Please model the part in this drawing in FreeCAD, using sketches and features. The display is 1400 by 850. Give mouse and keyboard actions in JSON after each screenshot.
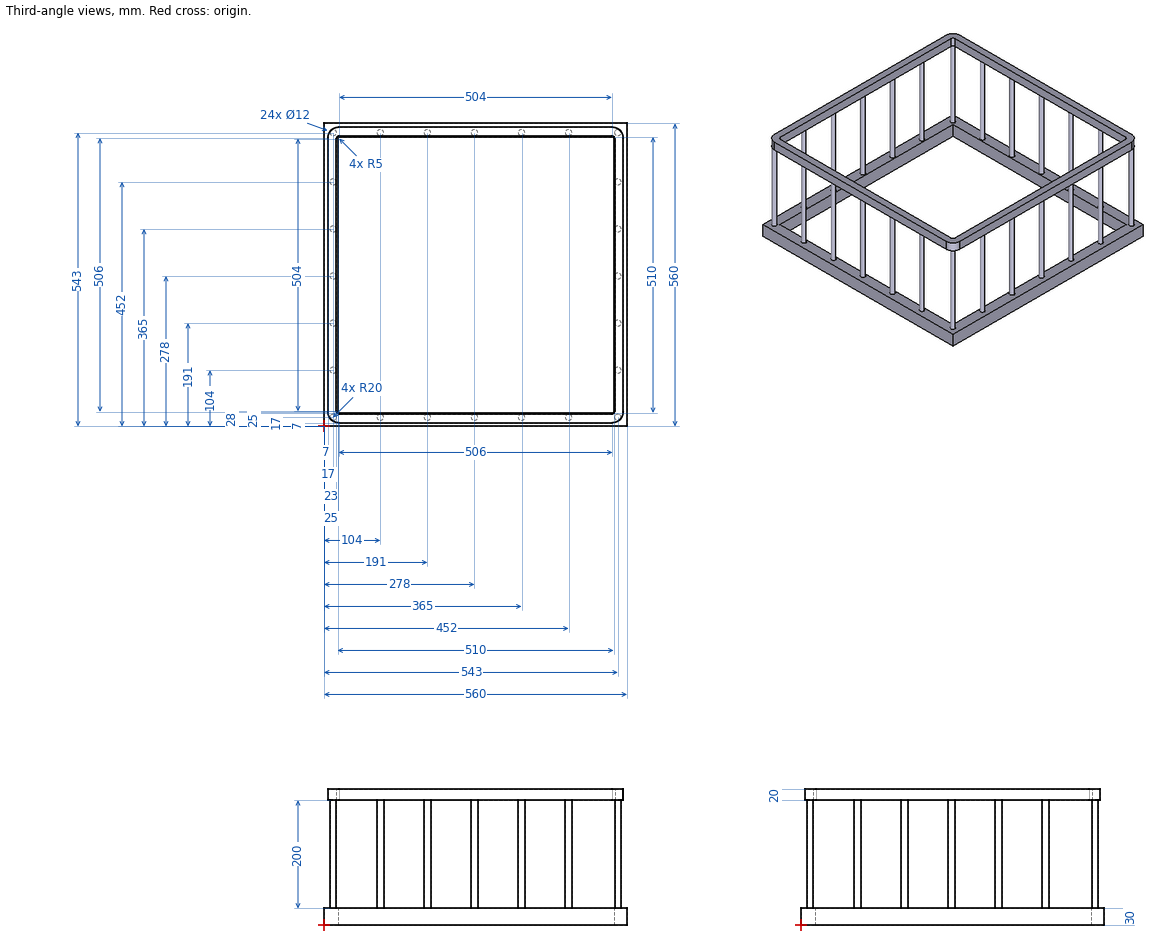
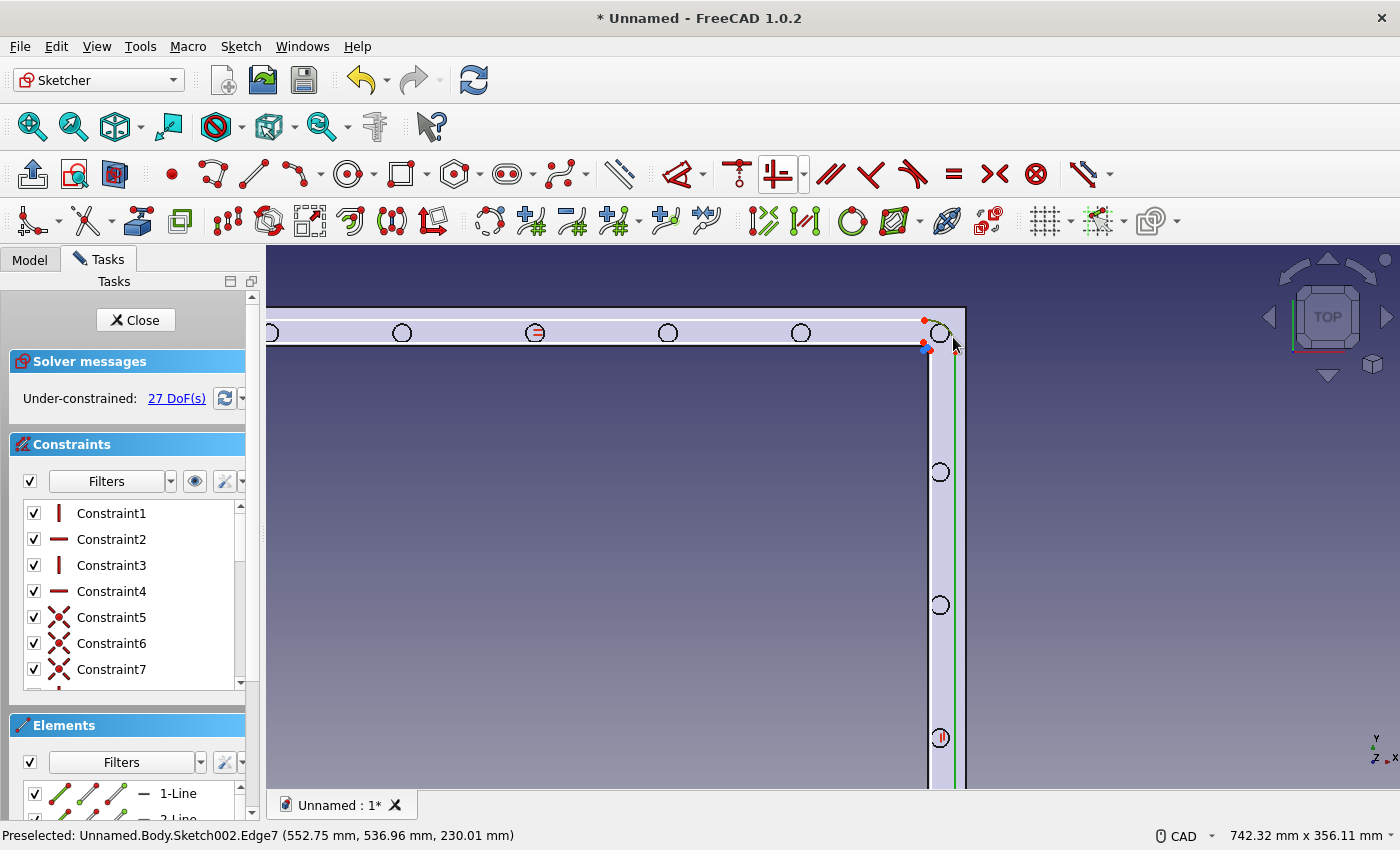
{"action": "left_click", "coordinate": [913, 174]}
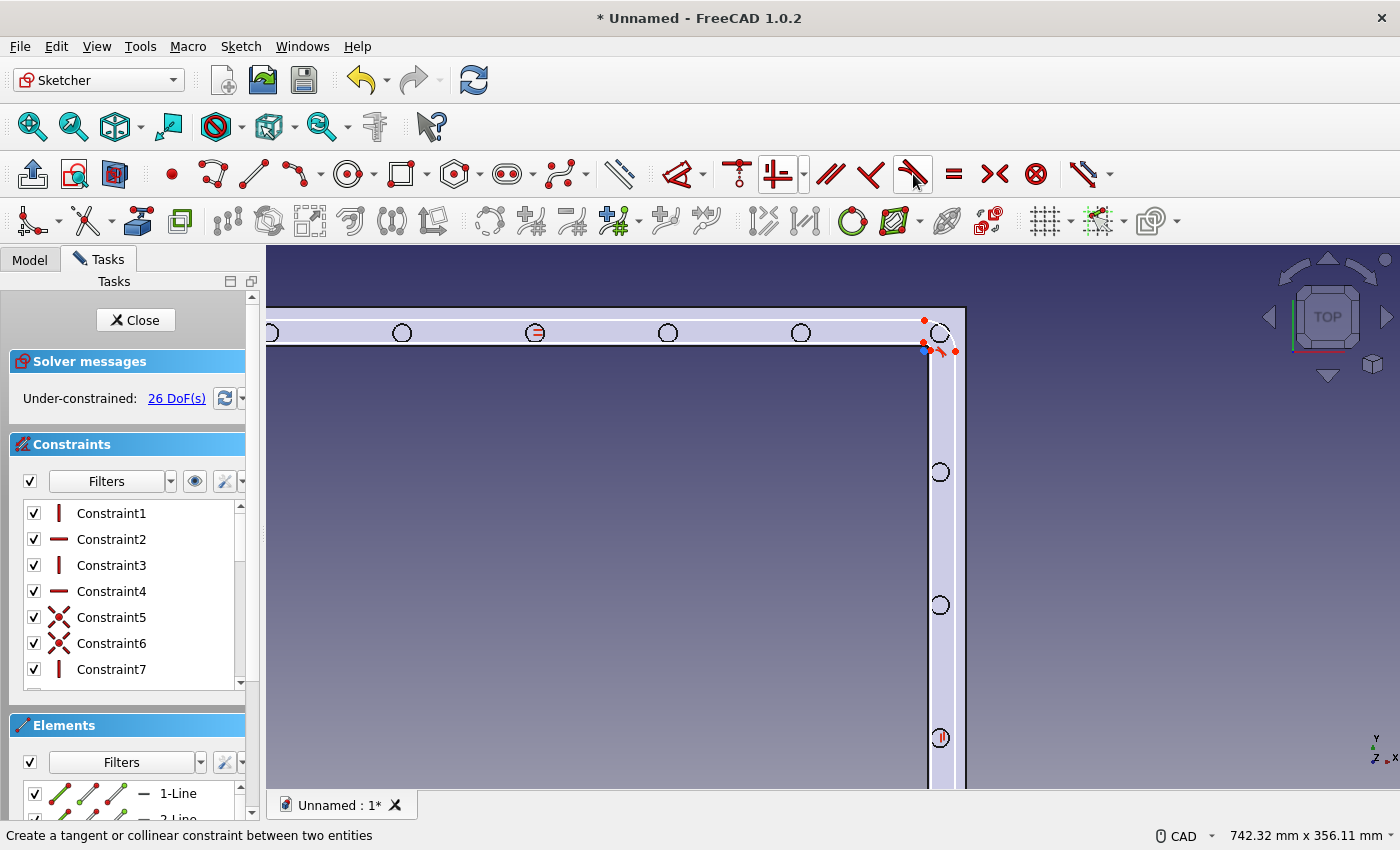
{"action": "left_click", "coordinate": [693, 320]}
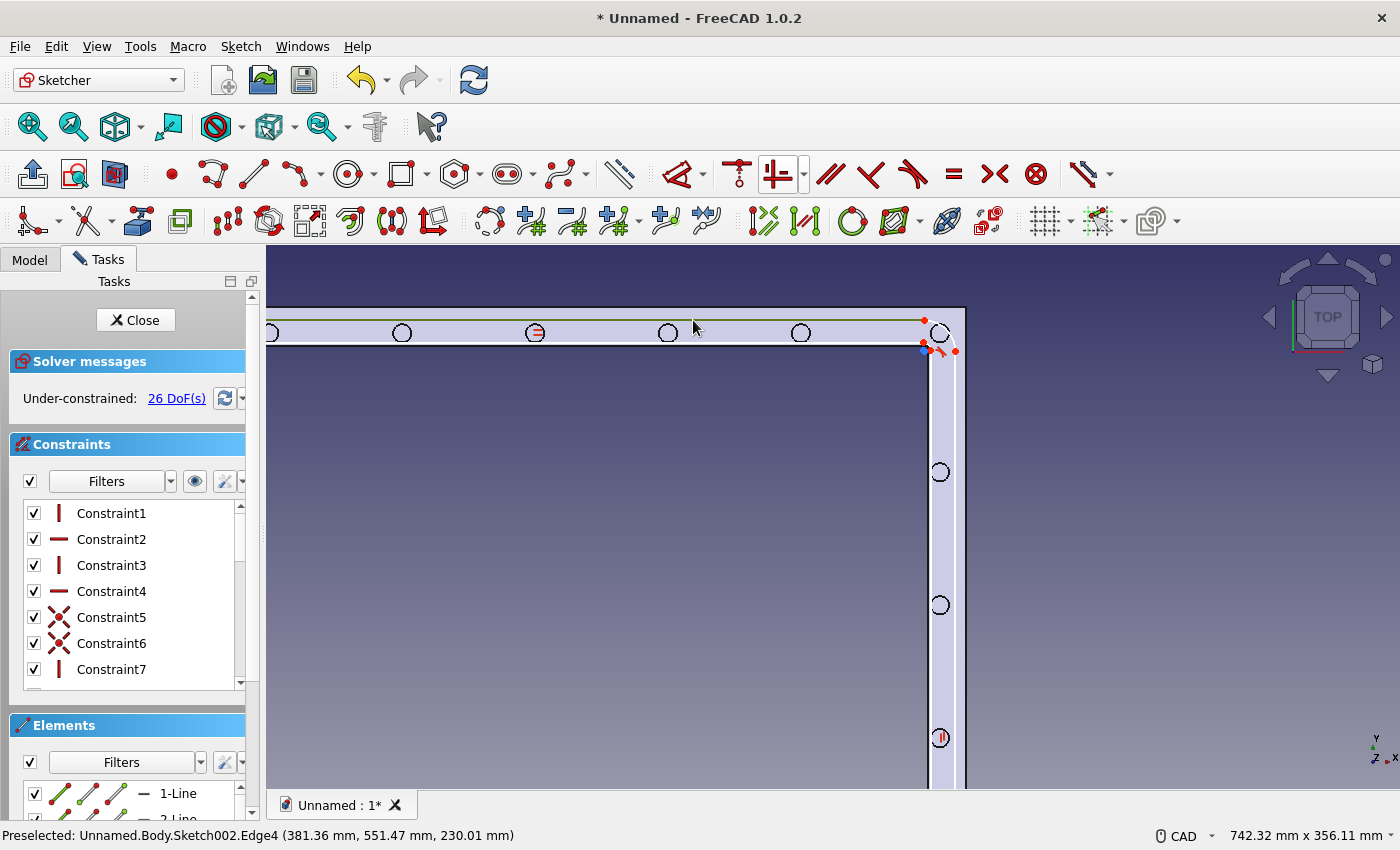
{"action": "left_click", "coordinate": [952, 338]}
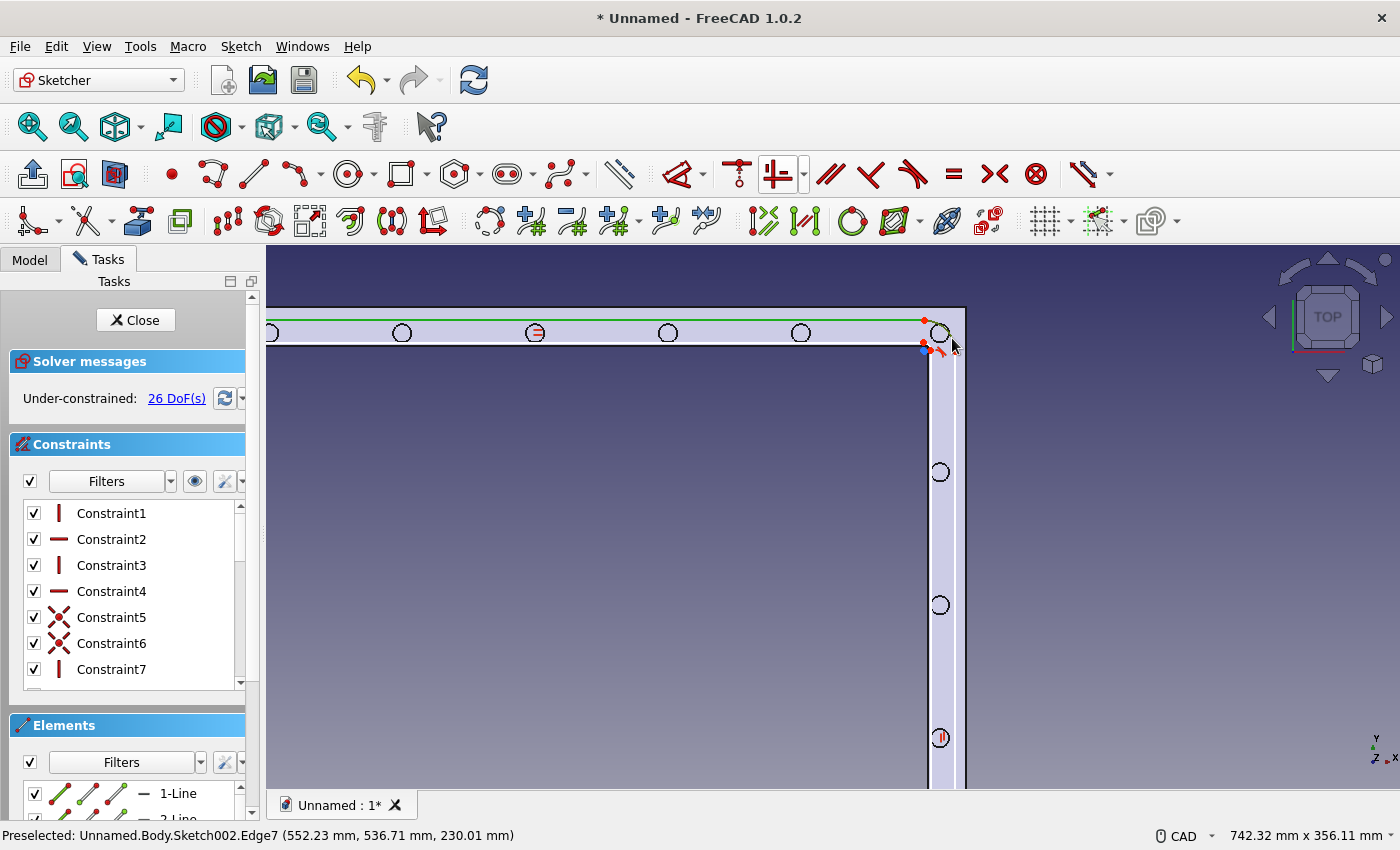
{"action": "left_click", "coordinate": [913, 174]}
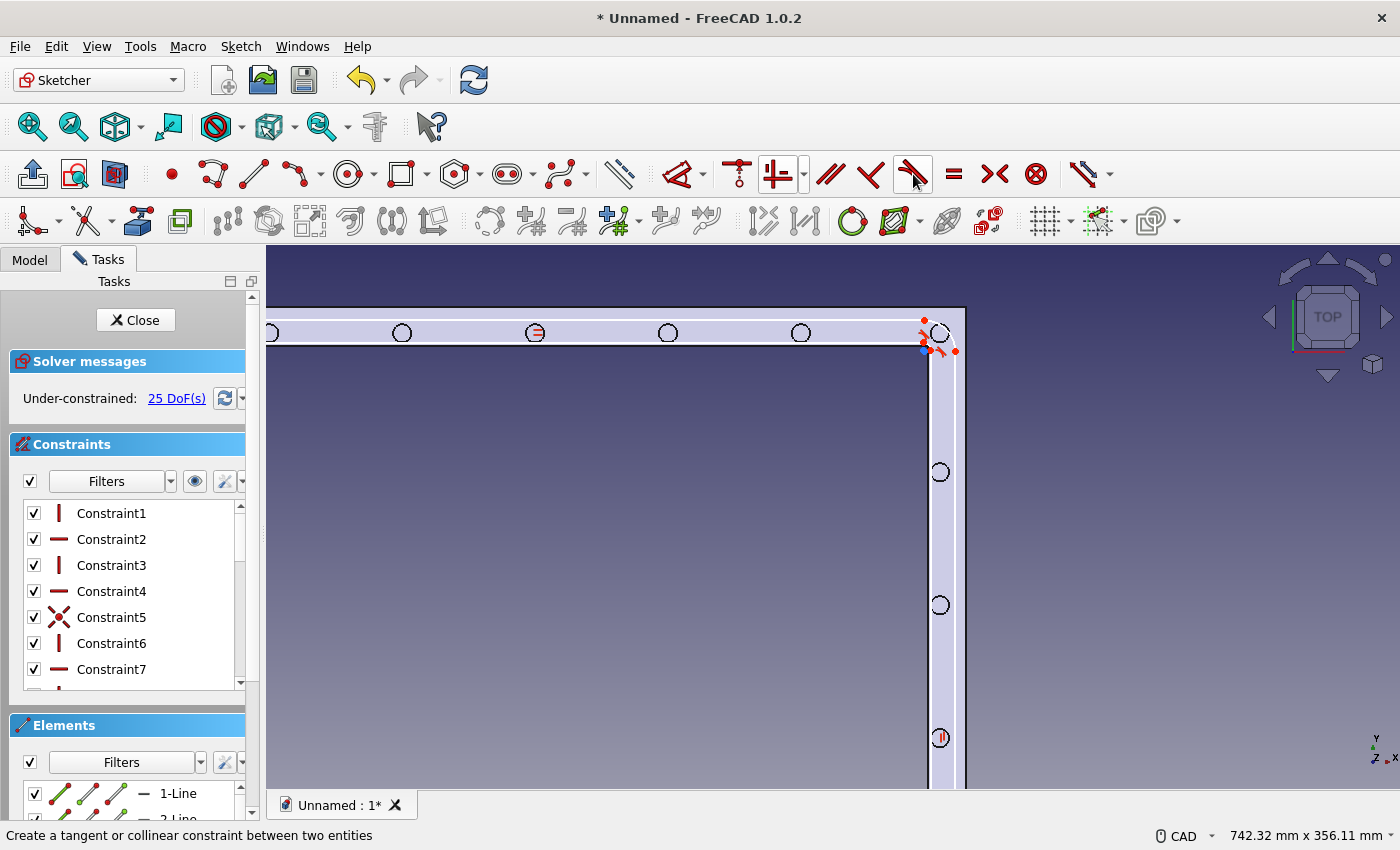
{"action": "left_click", "coordinate": [693, 320]}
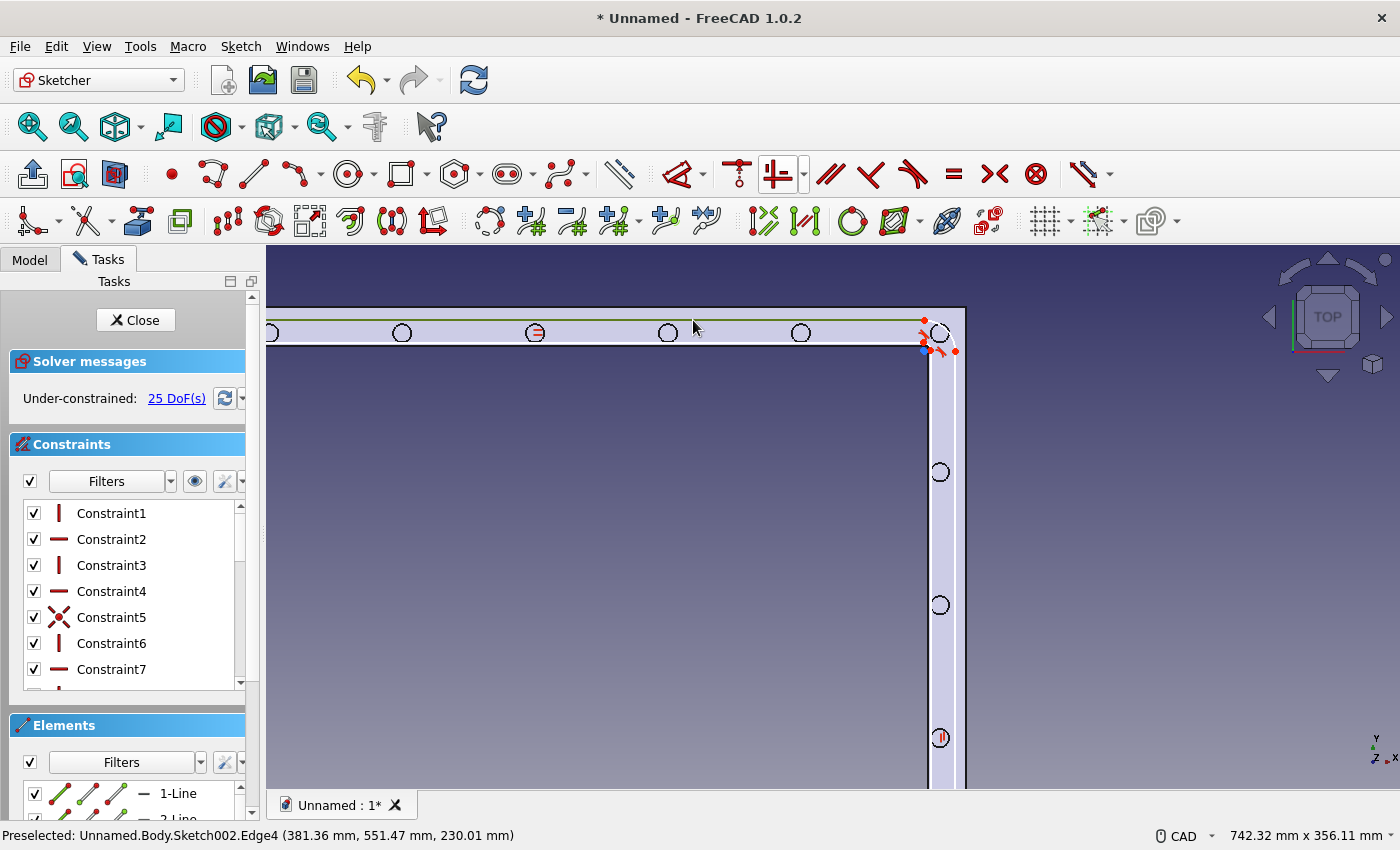
{"action": "scroll", "coordinate": [954, 335], "scroll_direction": "down", "scroll_amount": 4}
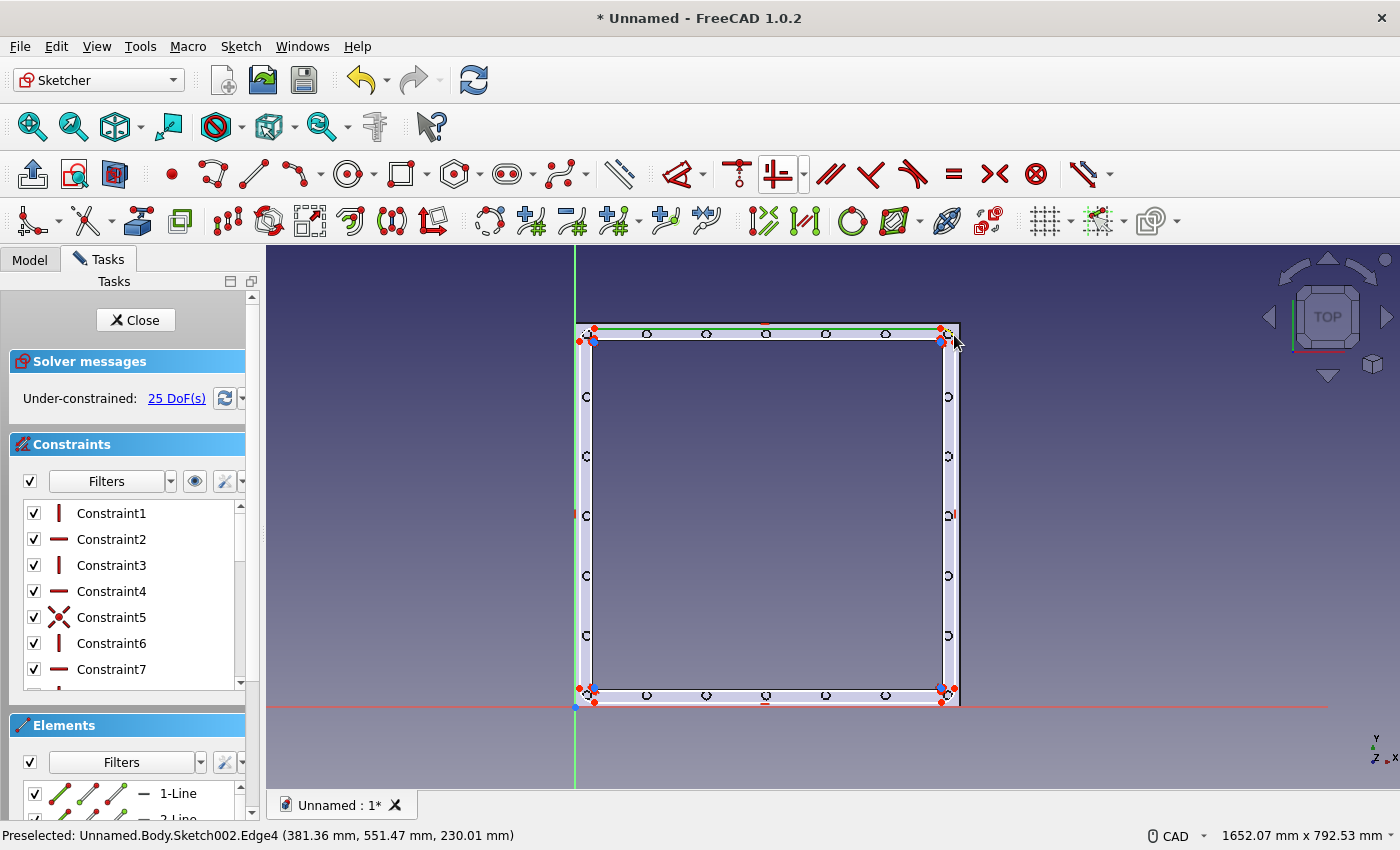
{"action": "scroll", "coordinate": [588, 330], "scroll_direction": "up", "scroll_amount": 4}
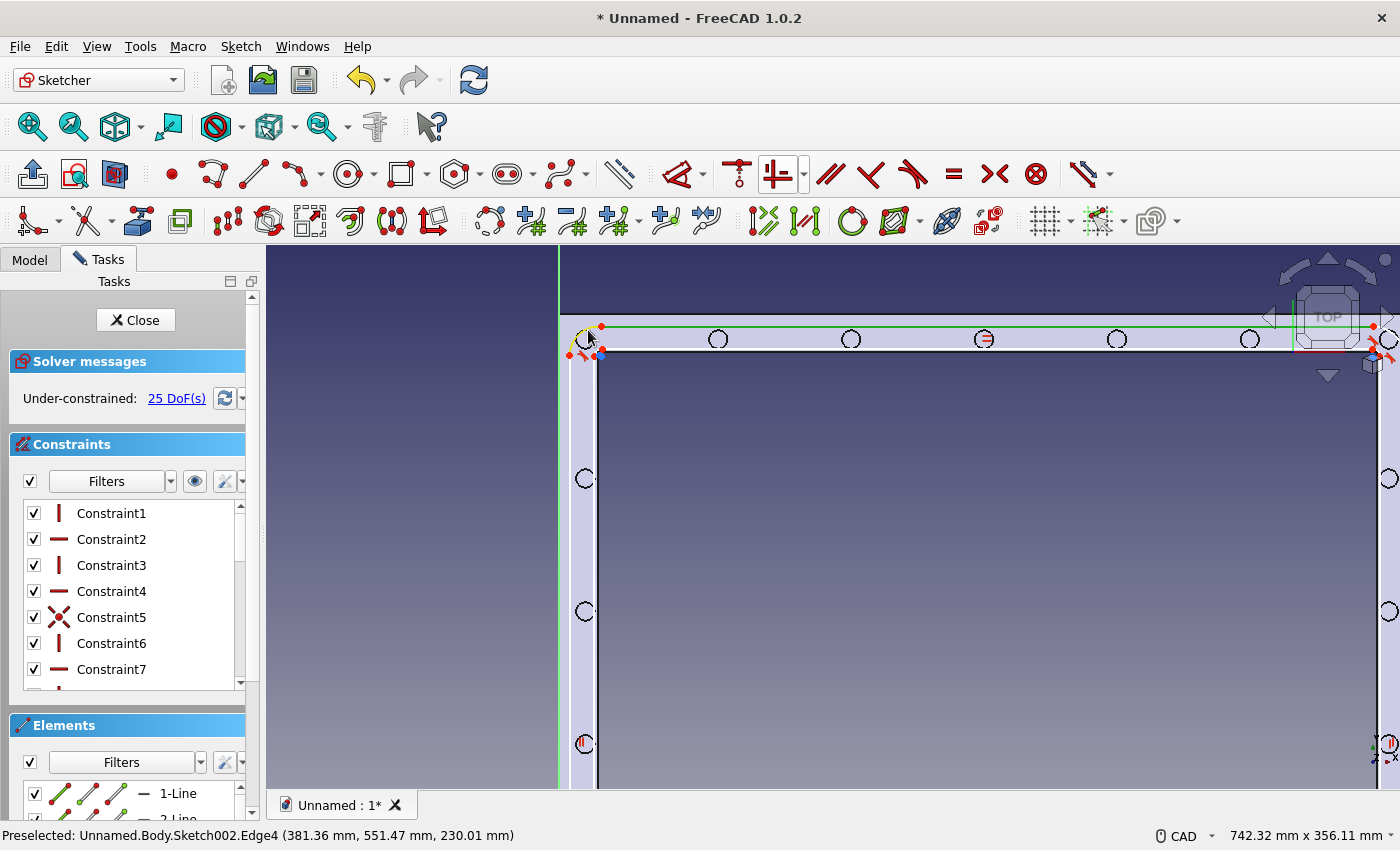
{"action": "left_click", "coordinate": [587, 329]}